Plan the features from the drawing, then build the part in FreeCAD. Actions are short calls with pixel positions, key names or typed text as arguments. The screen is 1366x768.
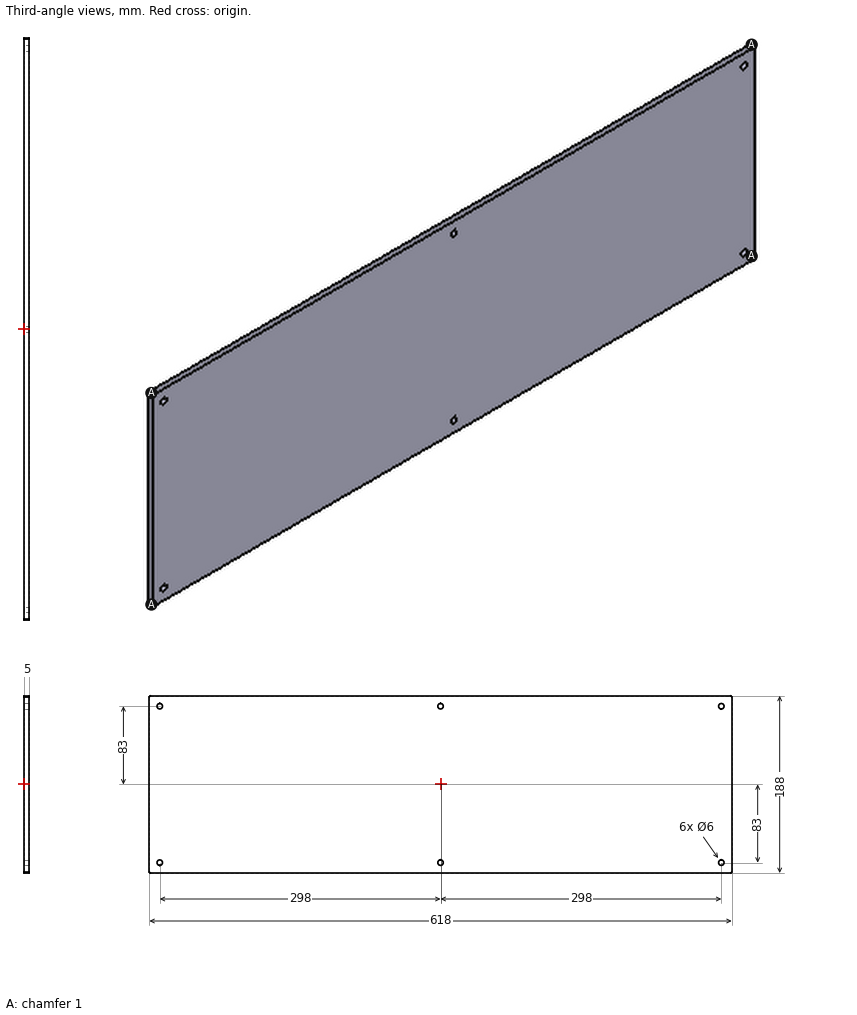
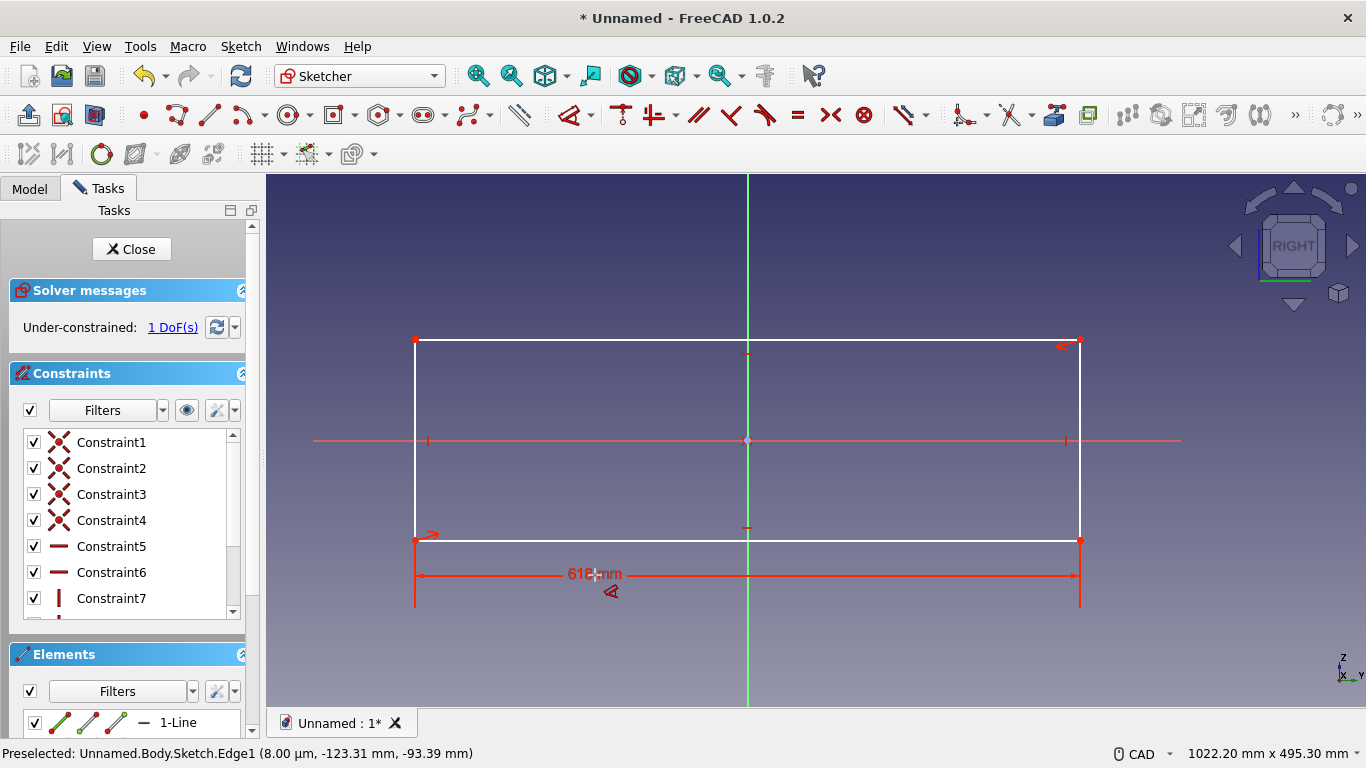
click(1080, 481)
click(1114, 394)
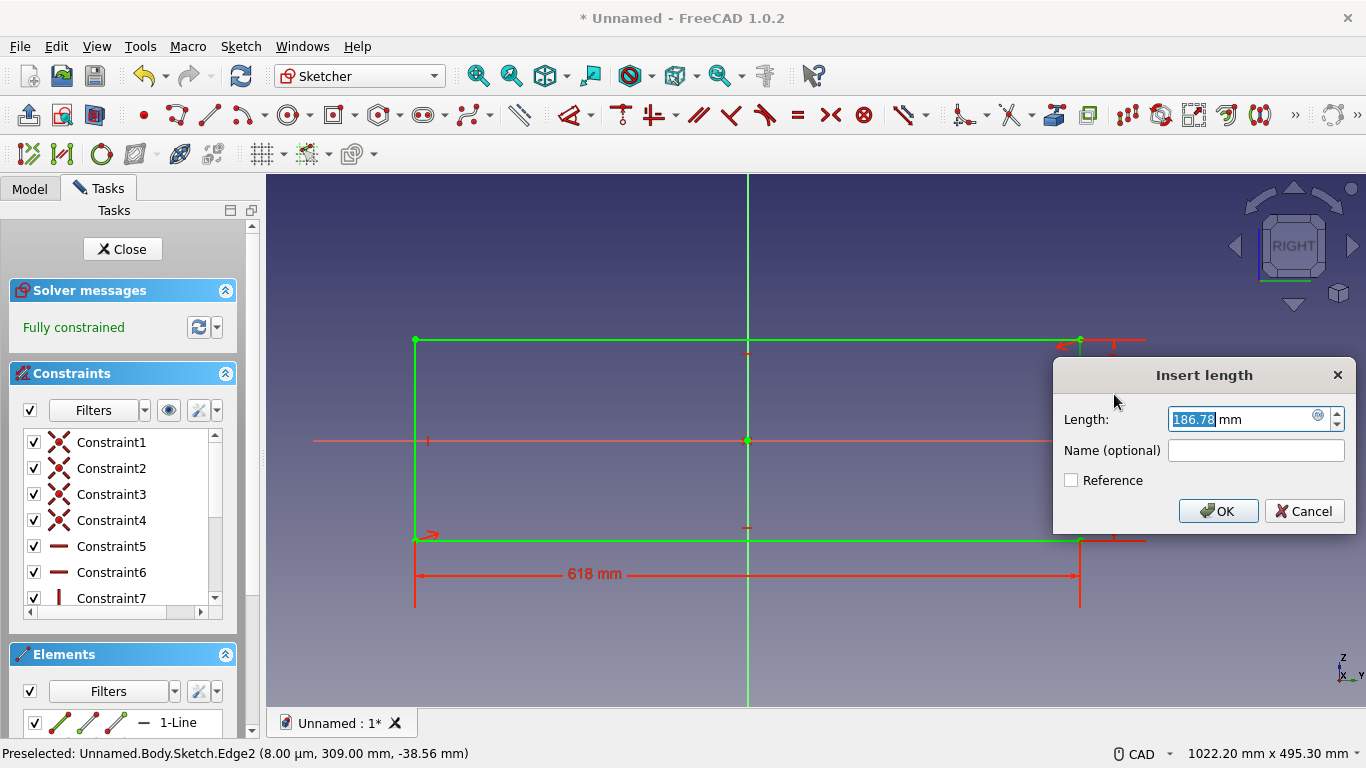
text(188)
key(Return)
key(Escape)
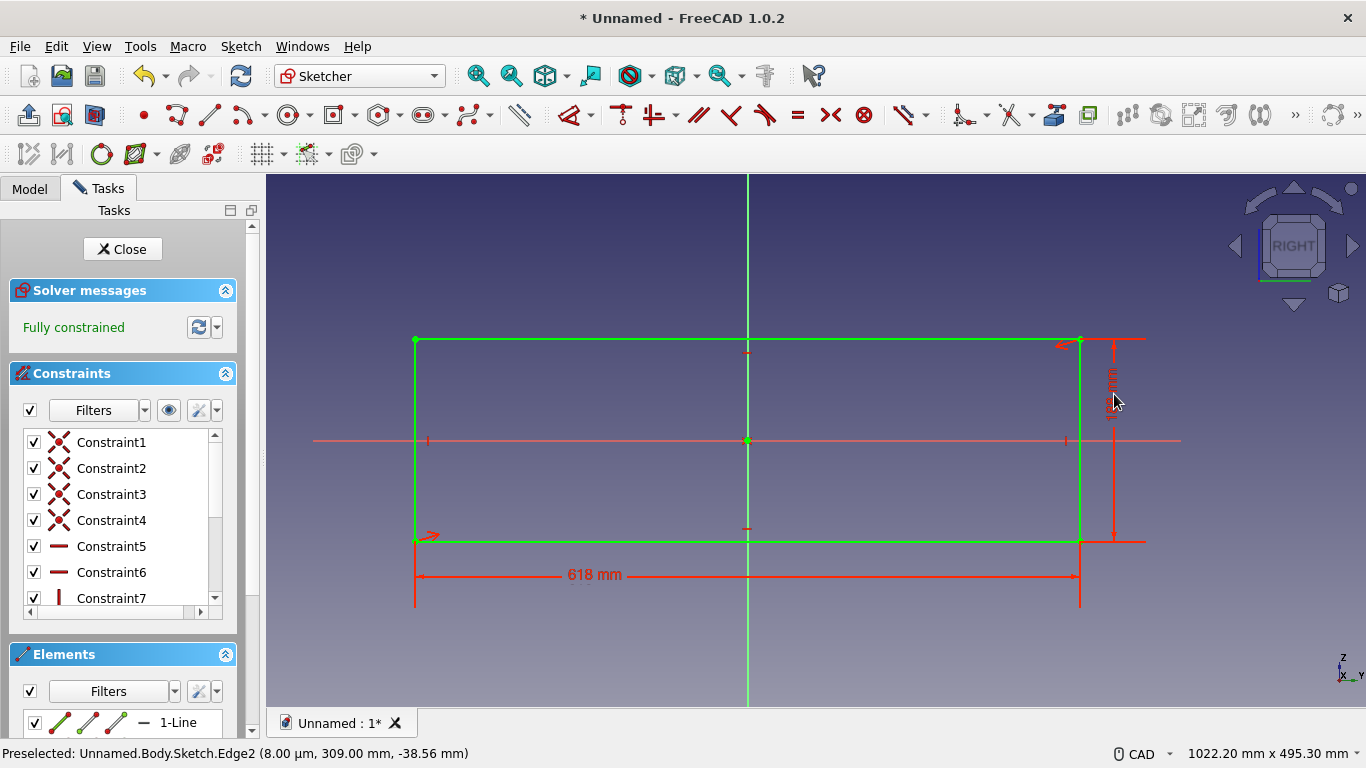
click(123, 249)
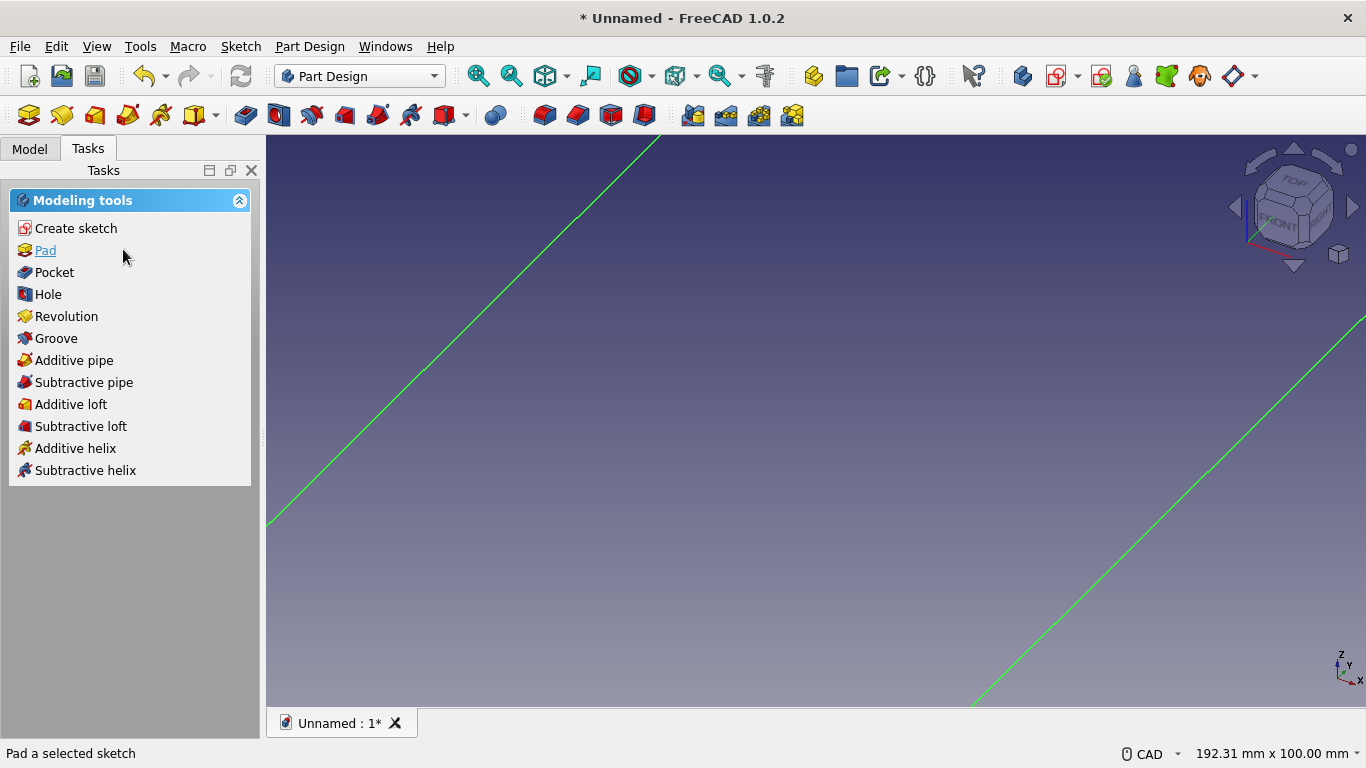
click(29, 116)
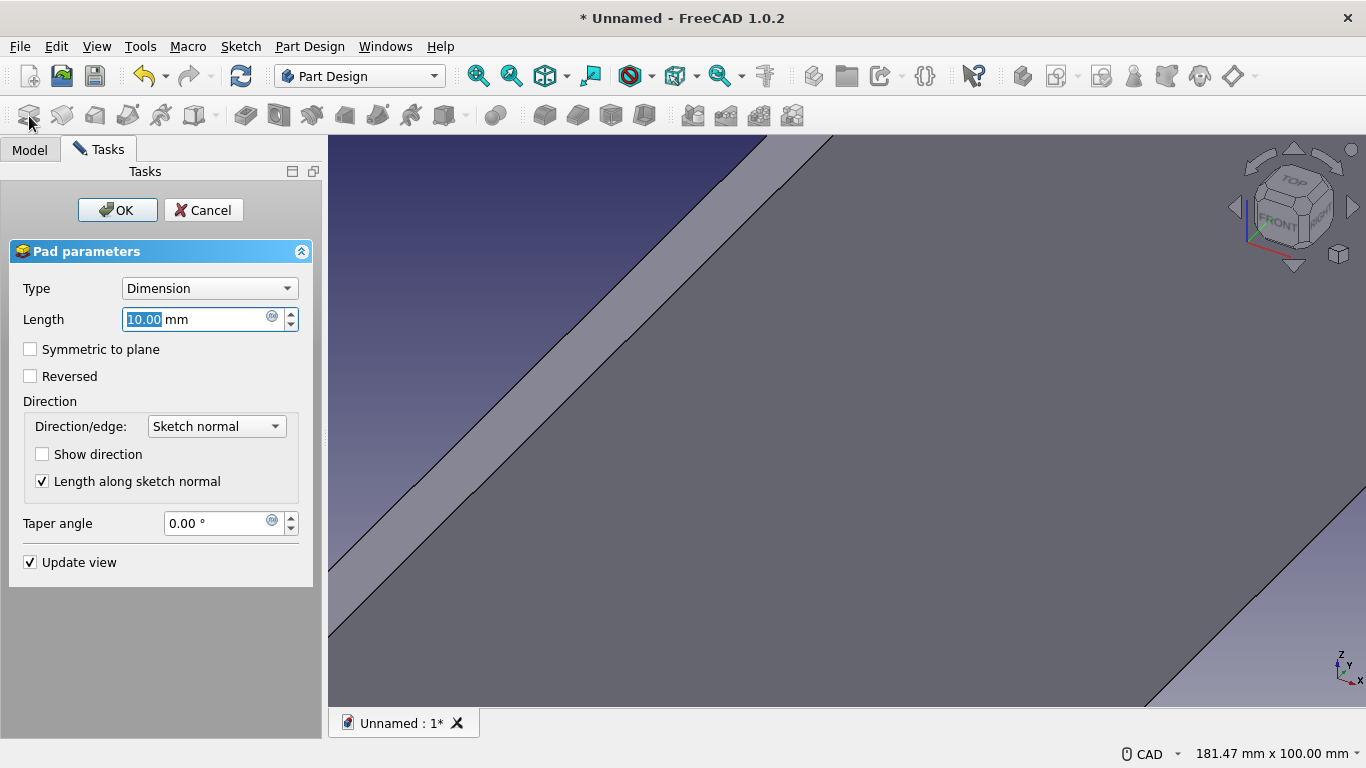
text(5)
key(Tab)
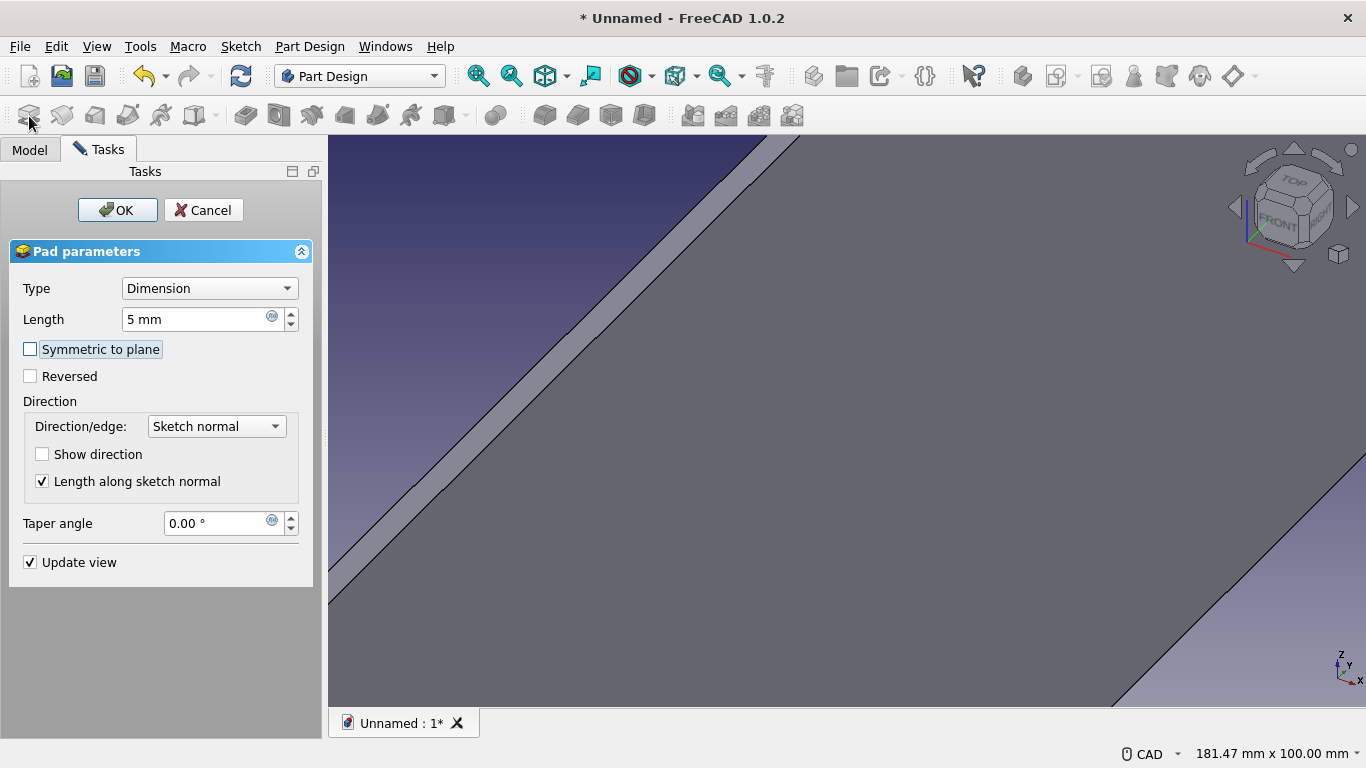
click(118, 210)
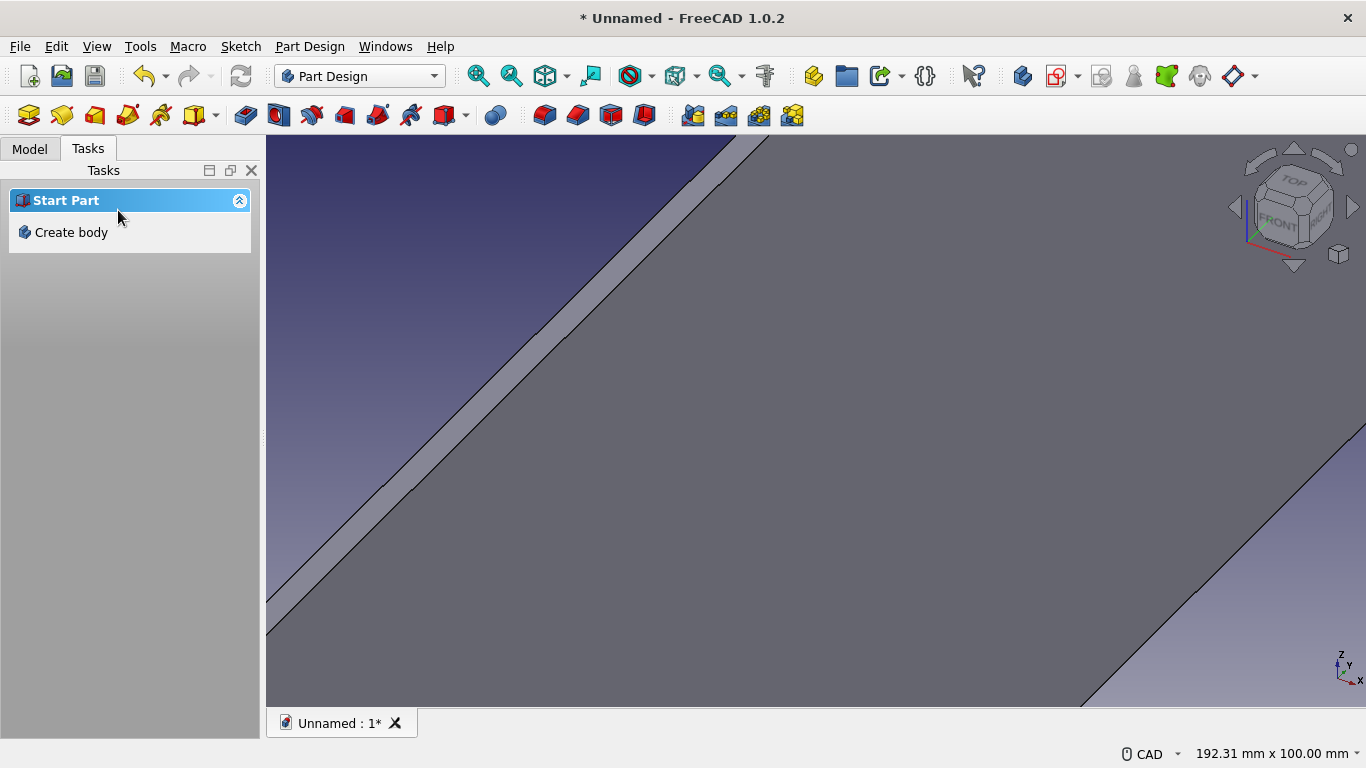
click(479, 76)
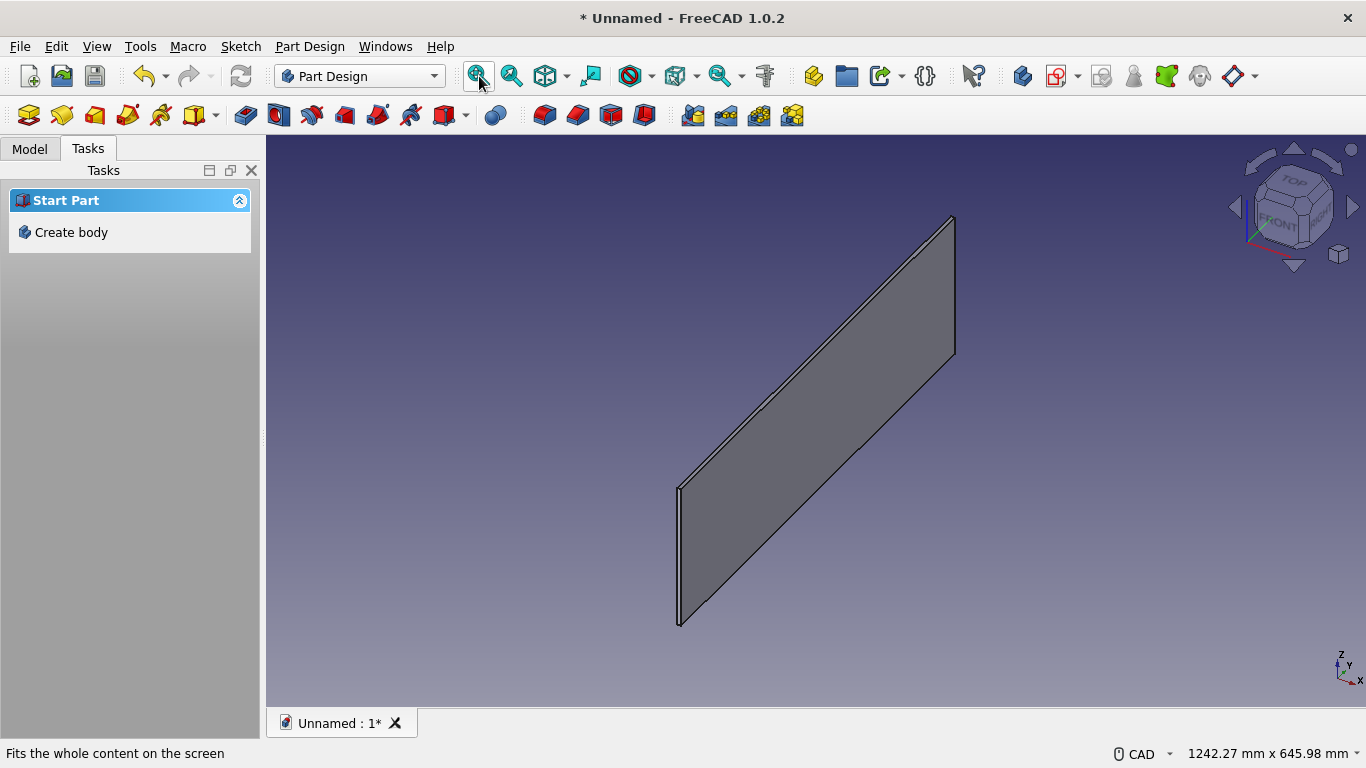
scroll(953, 216, up, 12)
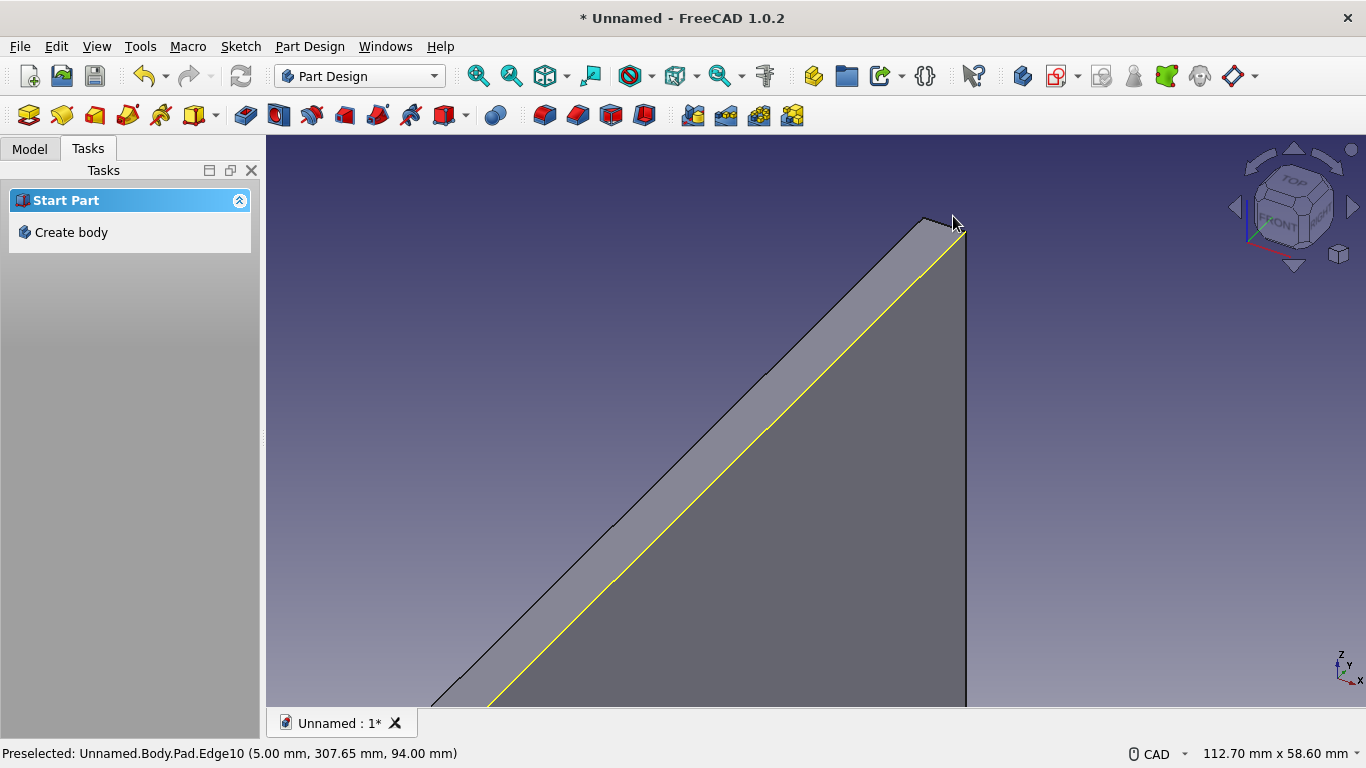
click(479, 76)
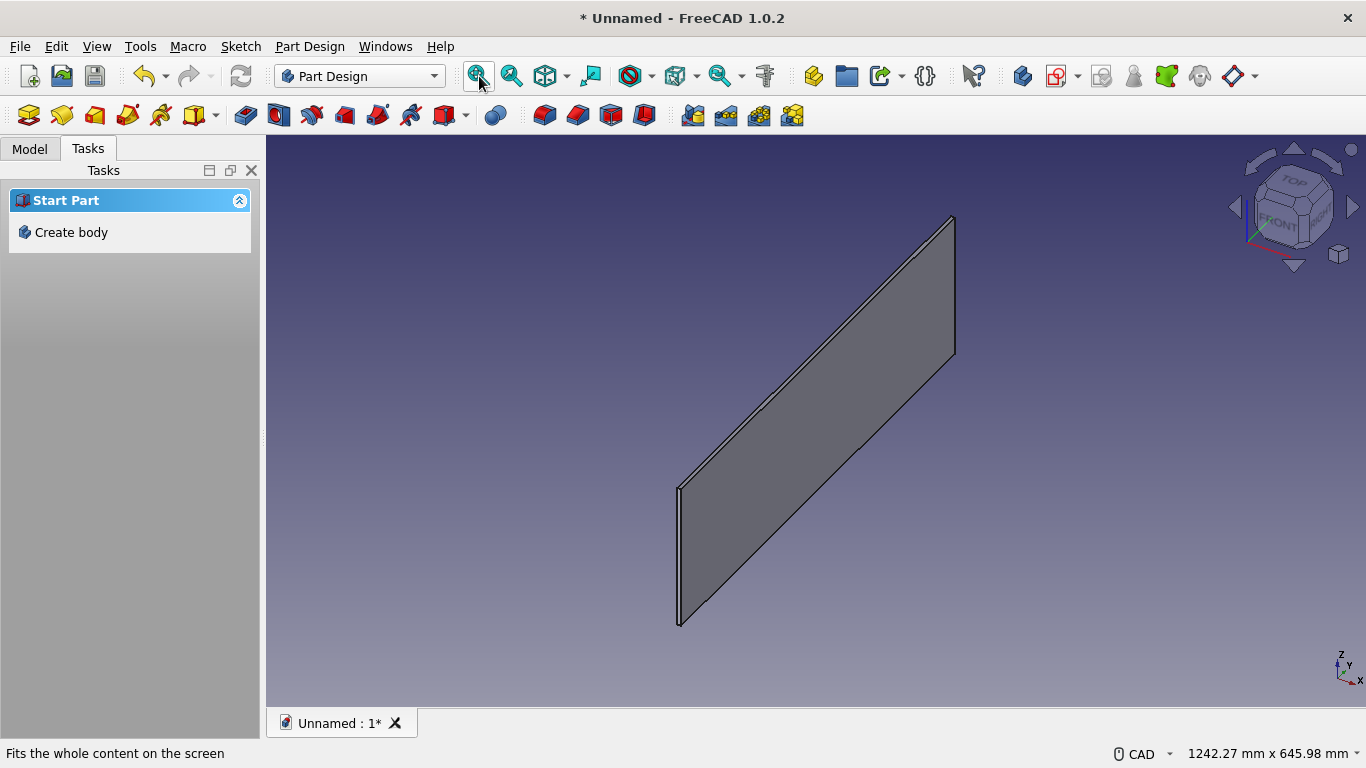
key(0)